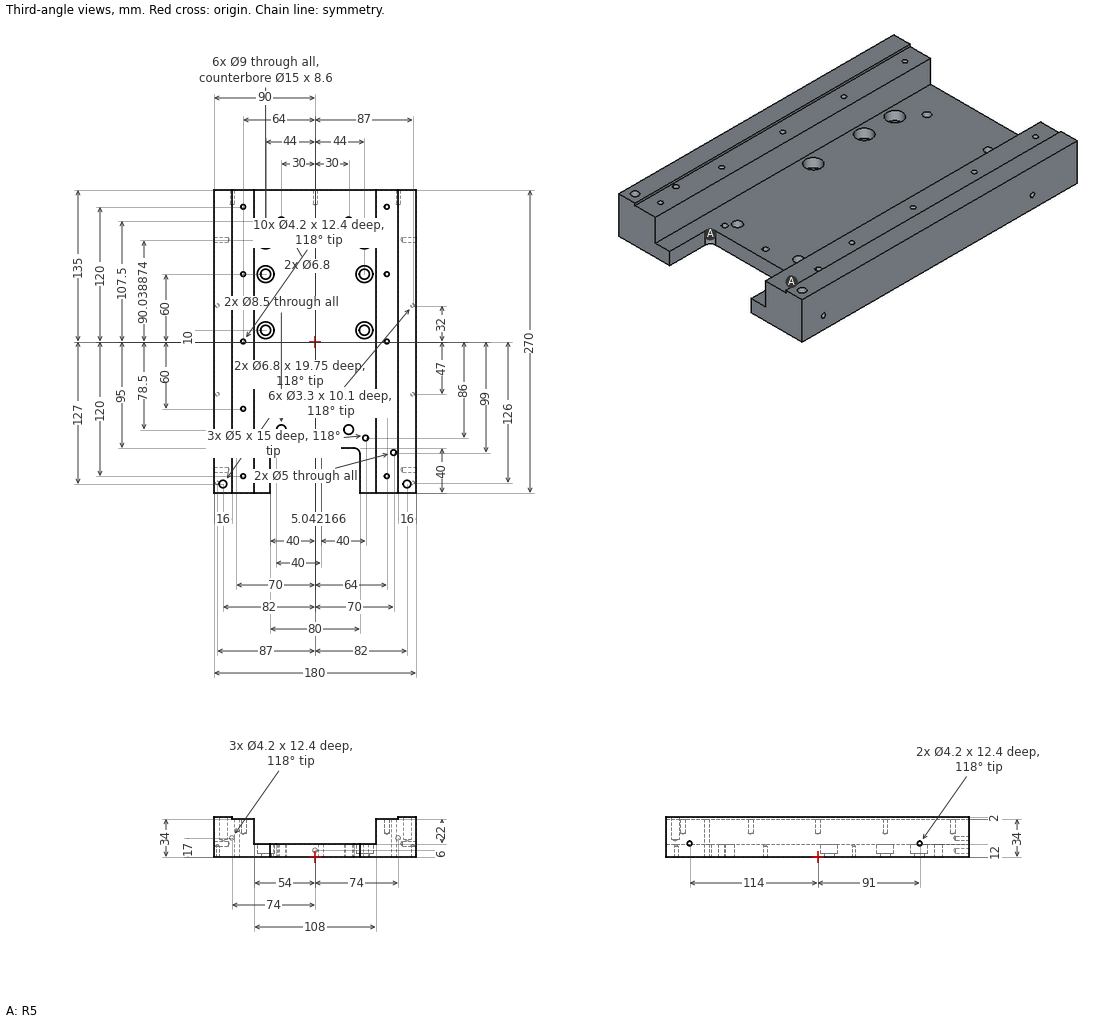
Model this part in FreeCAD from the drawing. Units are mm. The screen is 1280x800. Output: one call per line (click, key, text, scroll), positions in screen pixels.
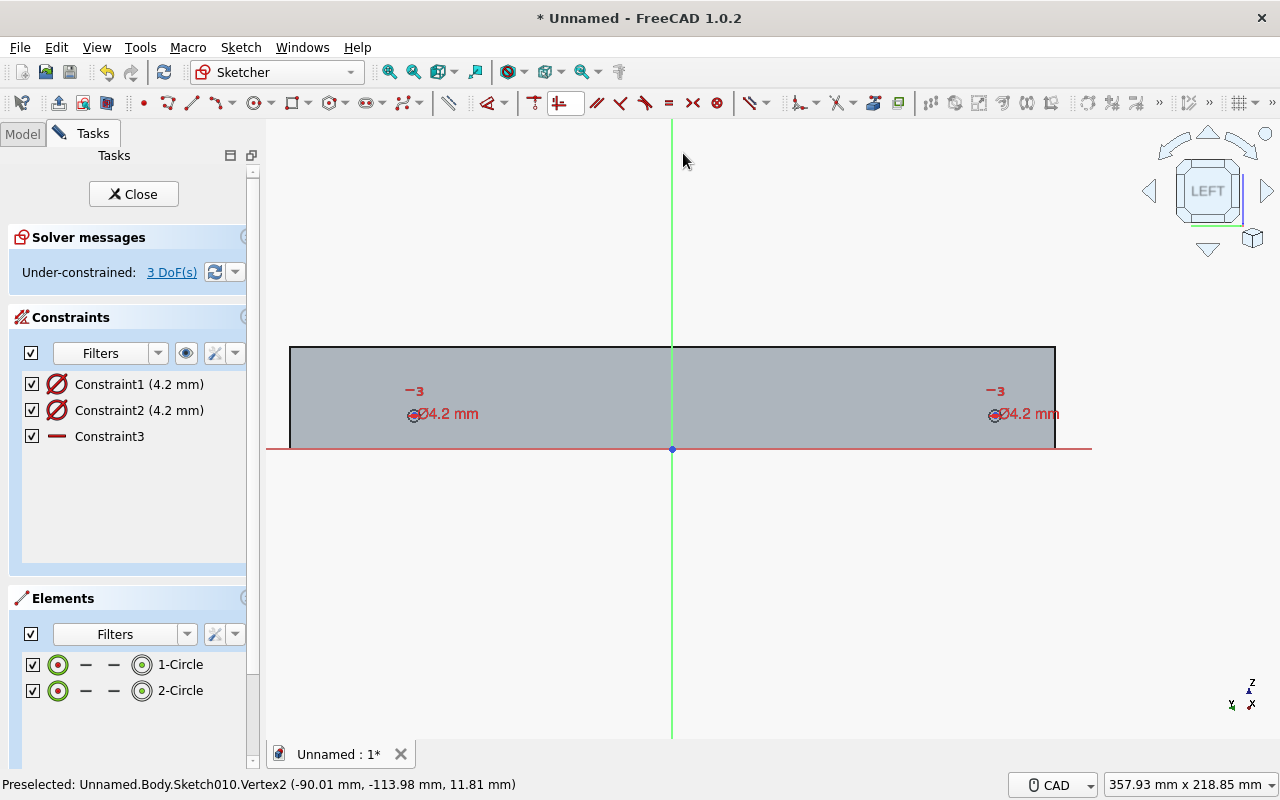
click(488, 104)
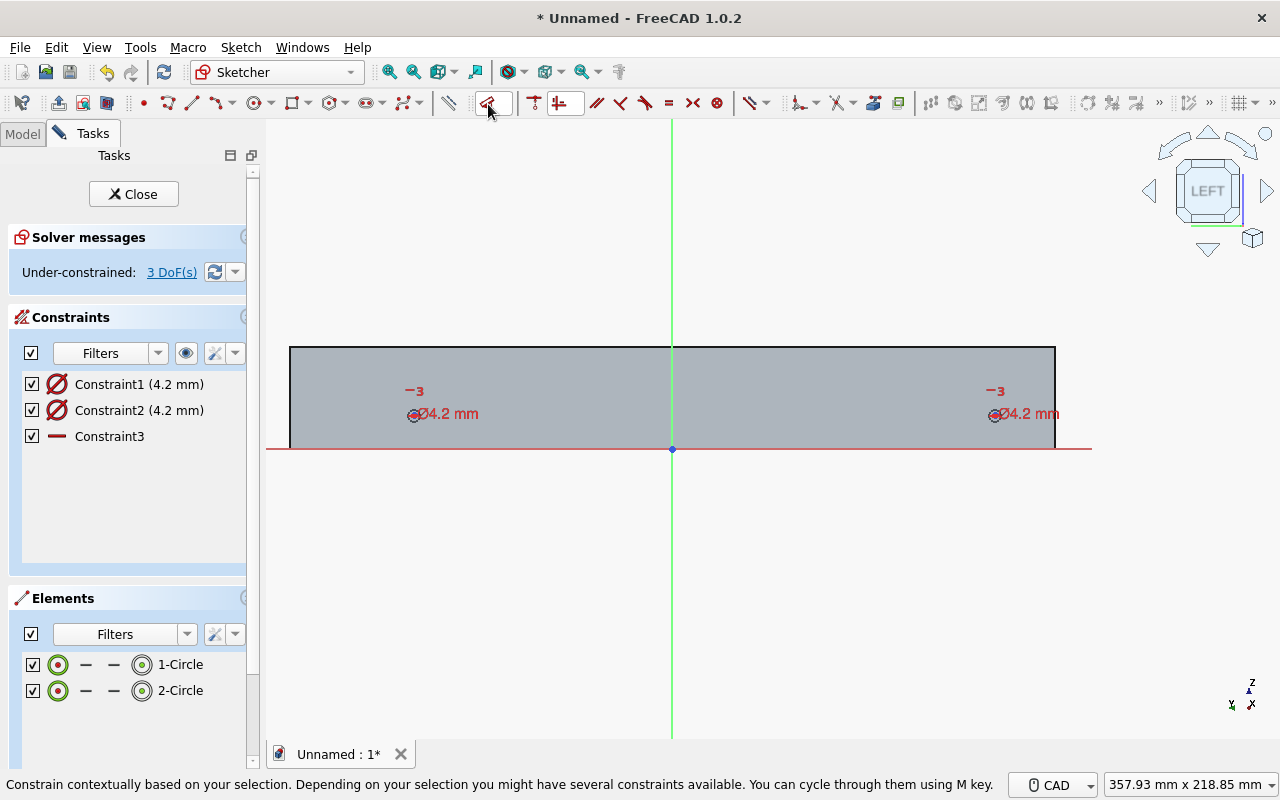
click(414, 416)
click(543, 483)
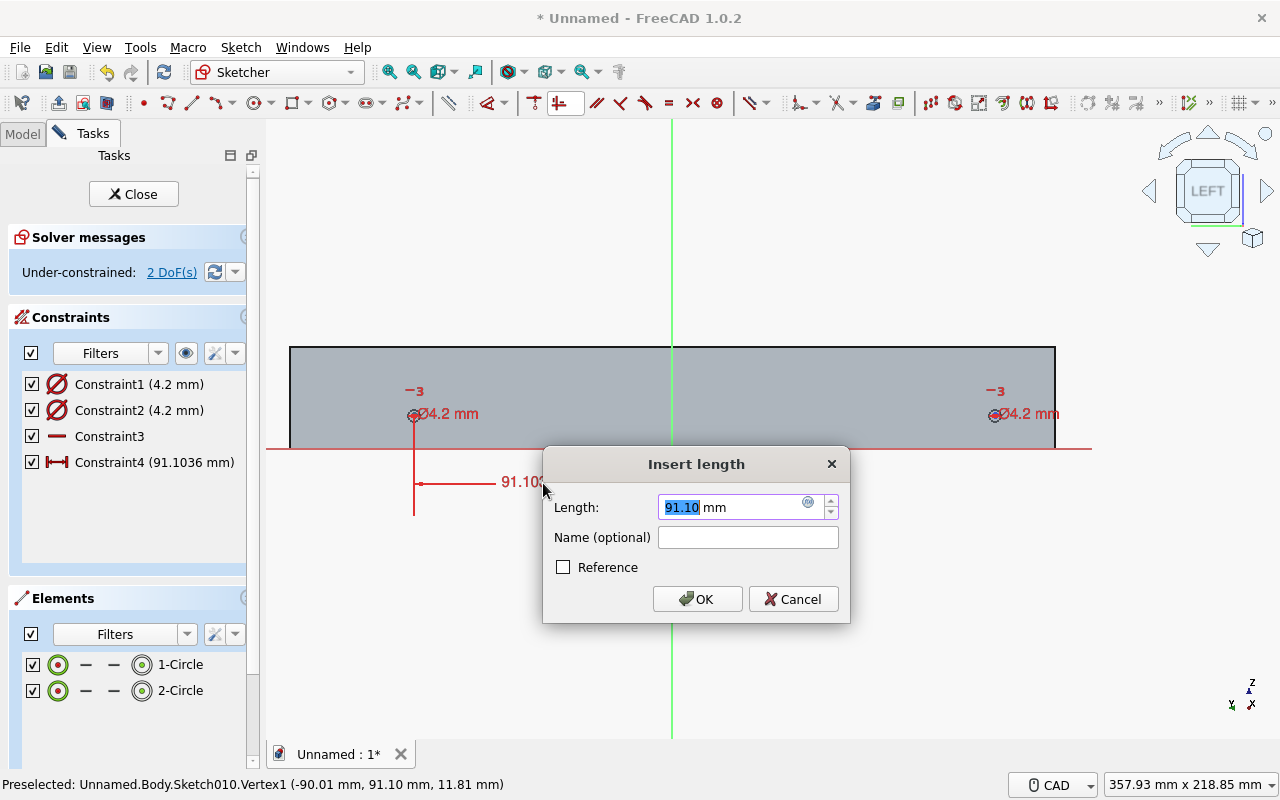
text(91)
key(Return)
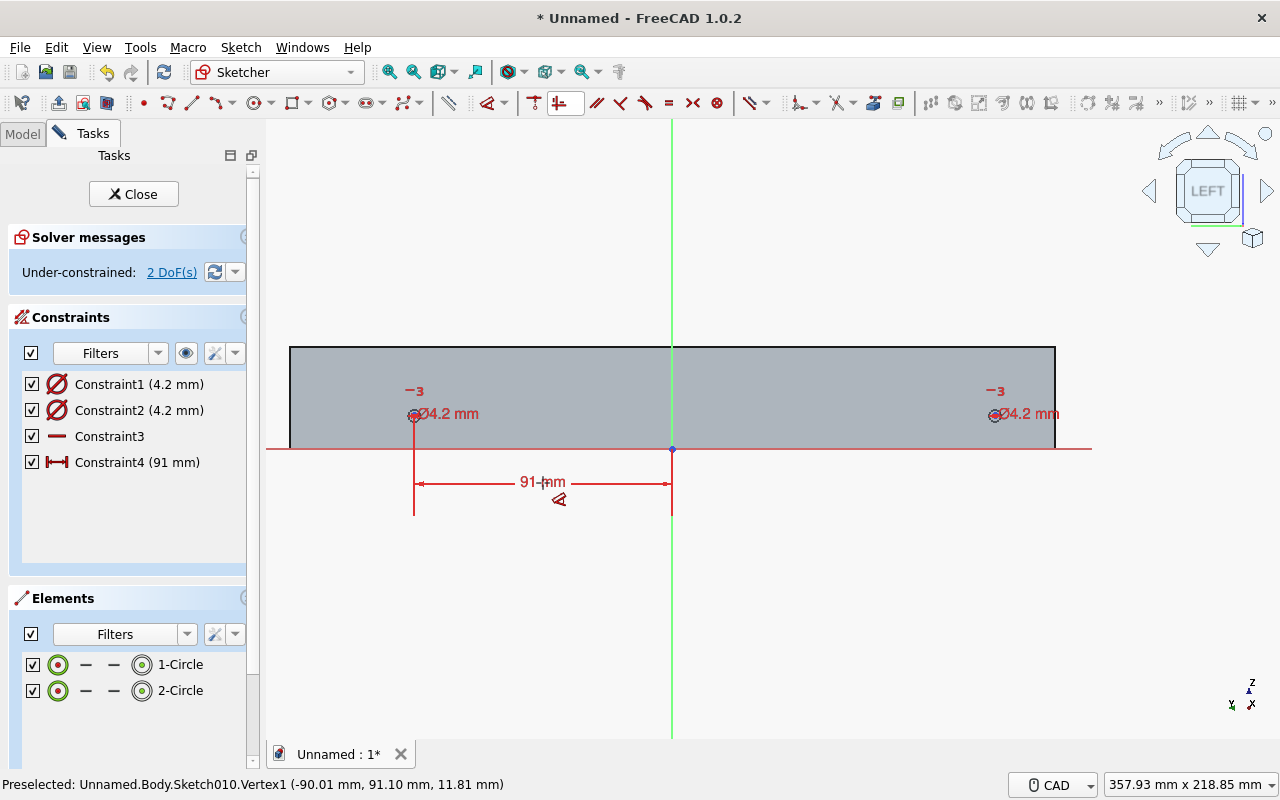
click(414, 416)
click(380, 433)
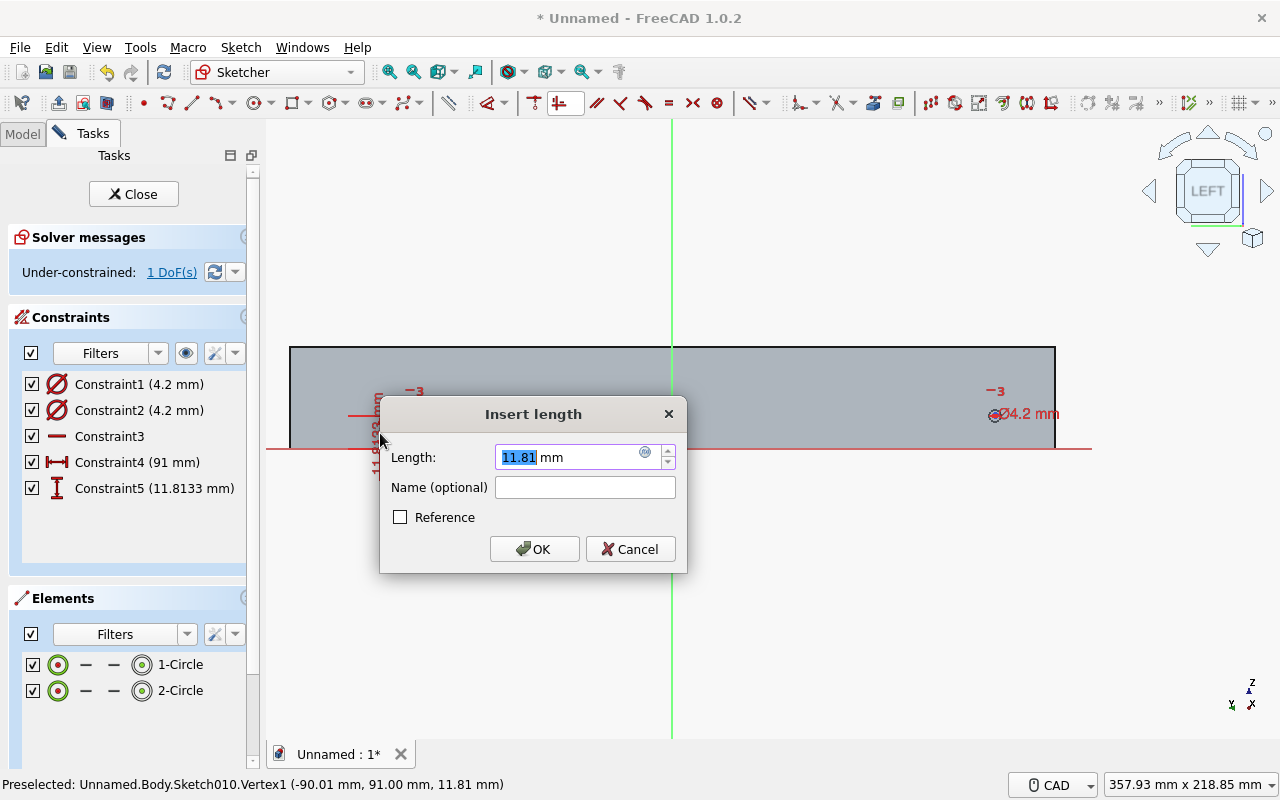
text(12)
key(Return)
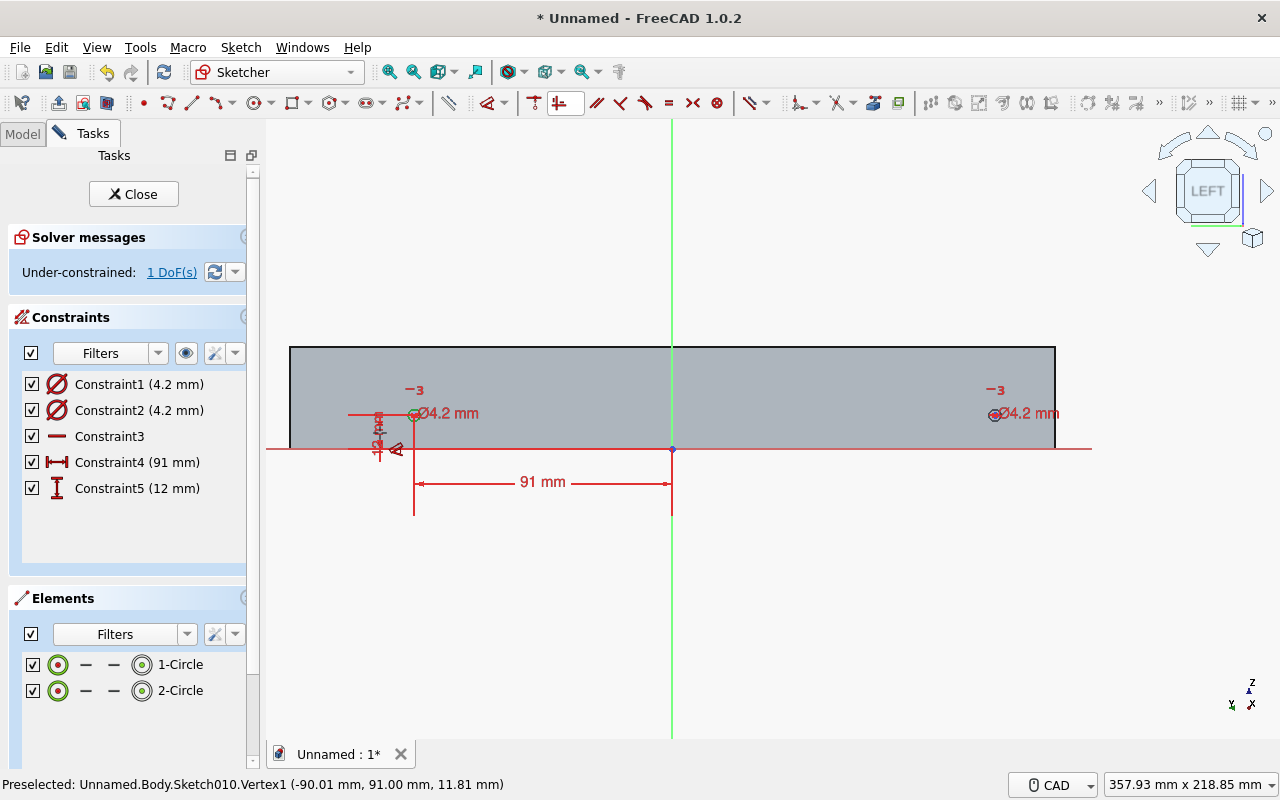
click(995, 415)
click(834, 483)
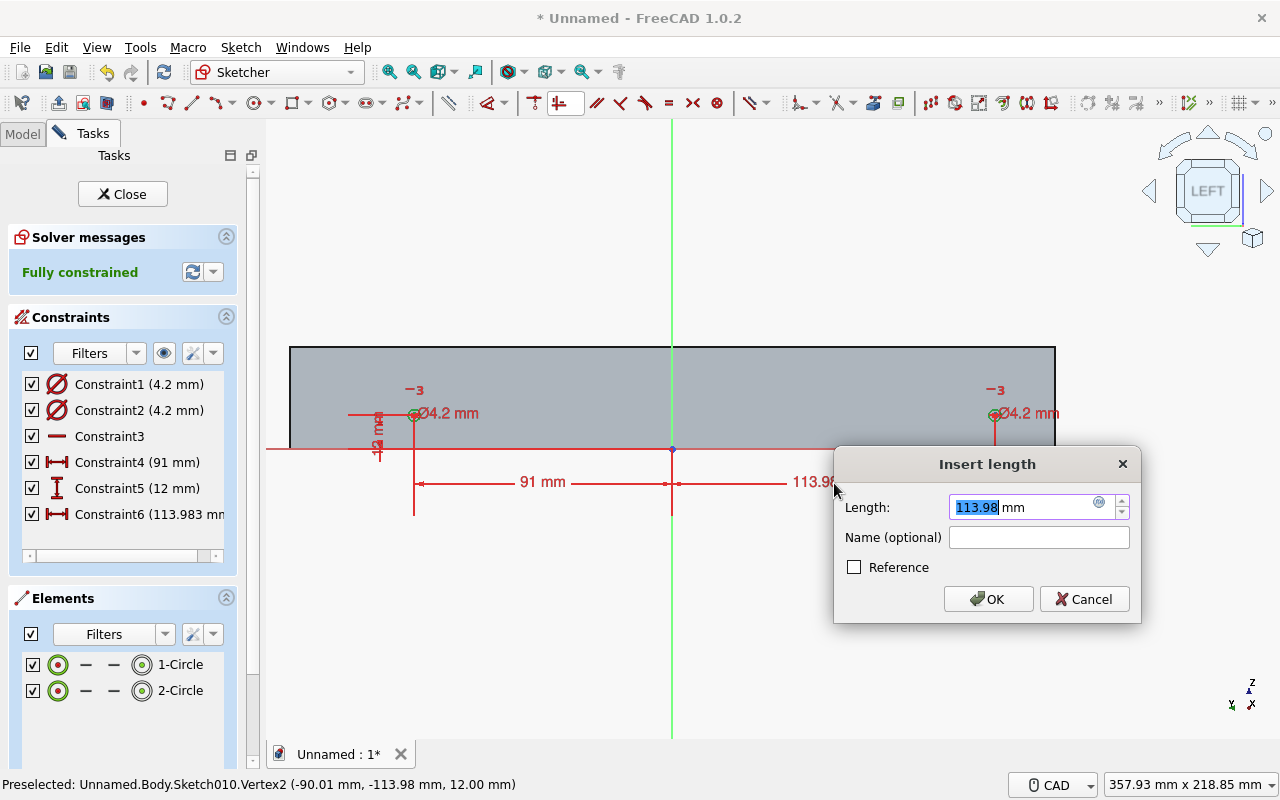
text(114)
key(Return)
key(Escape)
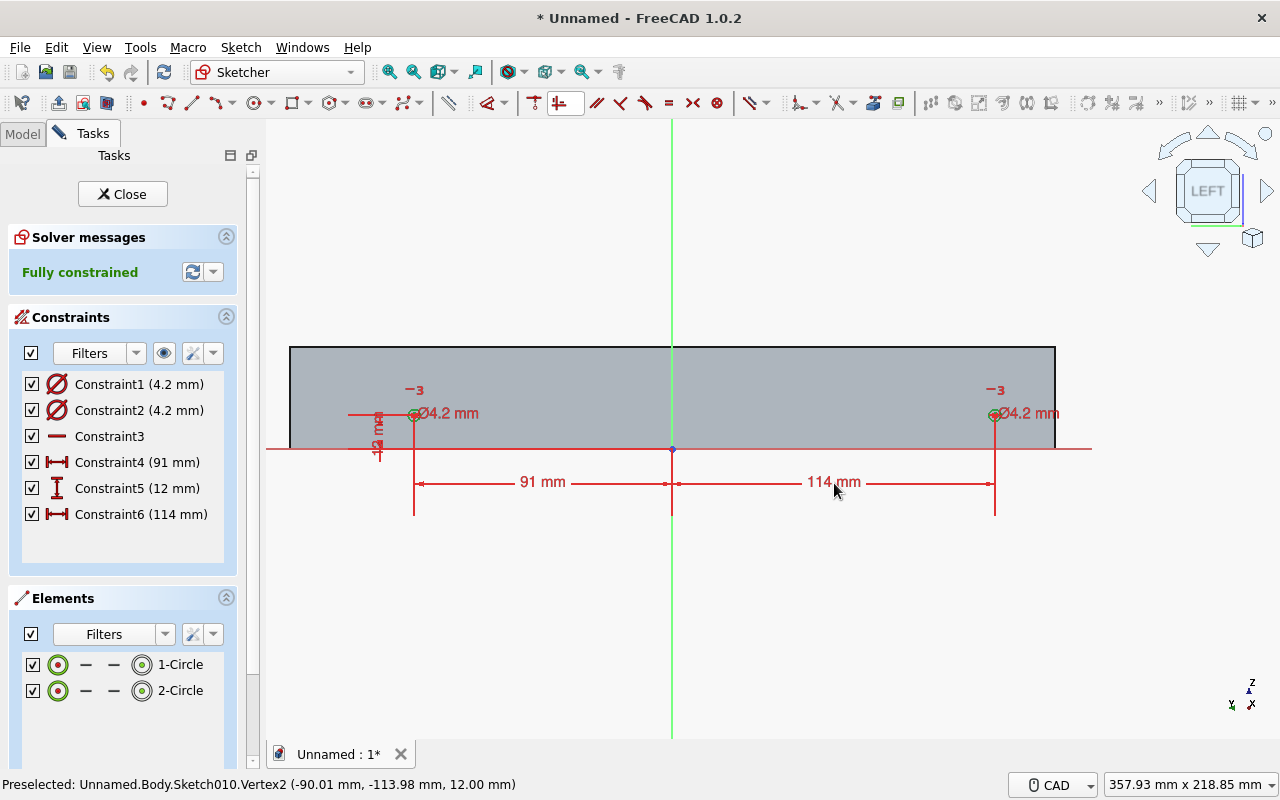
click(123, 194)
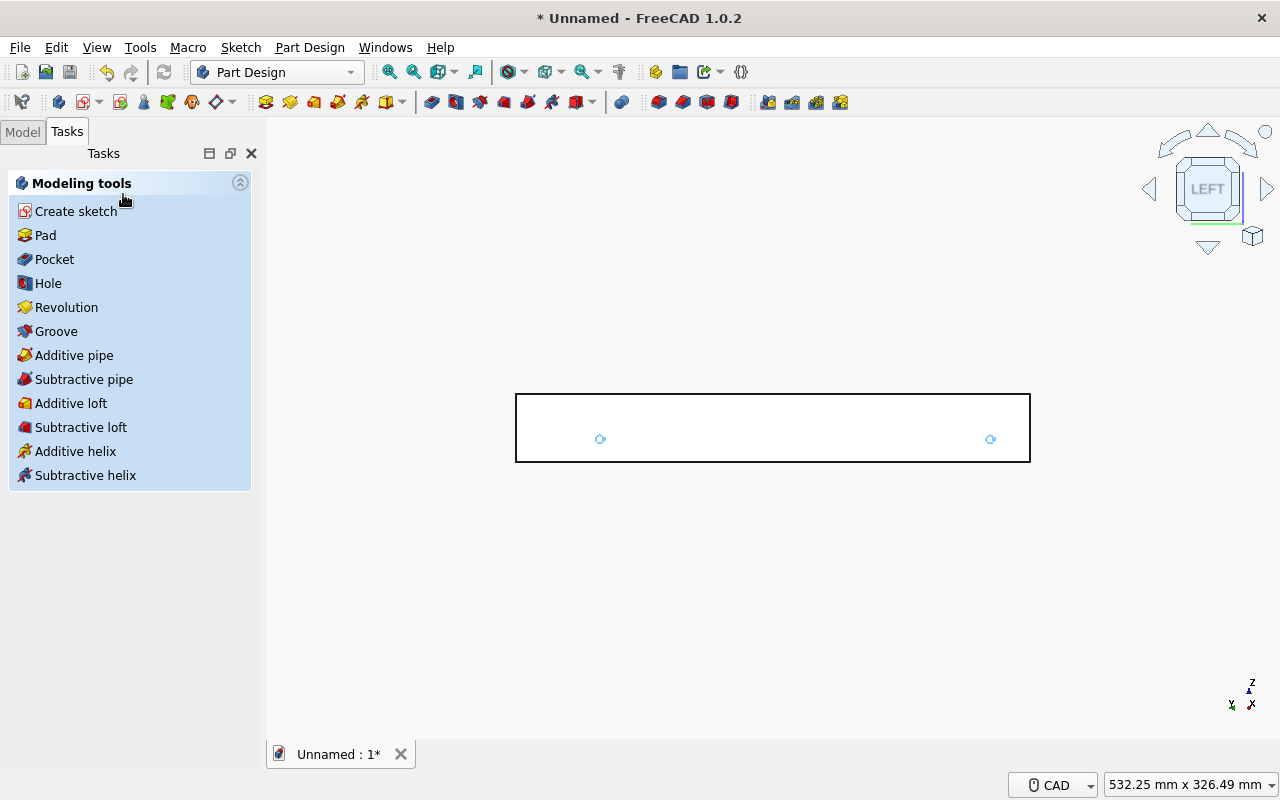
click(456, 102)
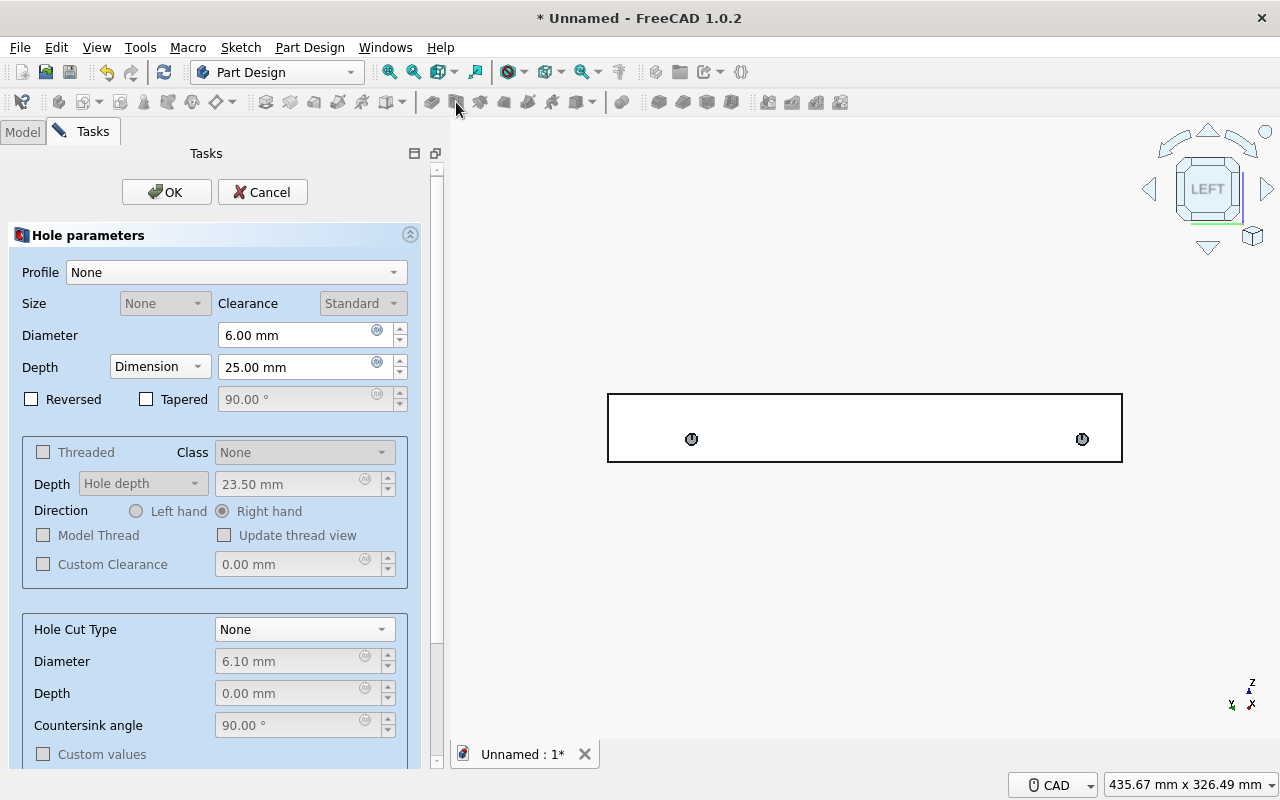
triple_click(305, 335)